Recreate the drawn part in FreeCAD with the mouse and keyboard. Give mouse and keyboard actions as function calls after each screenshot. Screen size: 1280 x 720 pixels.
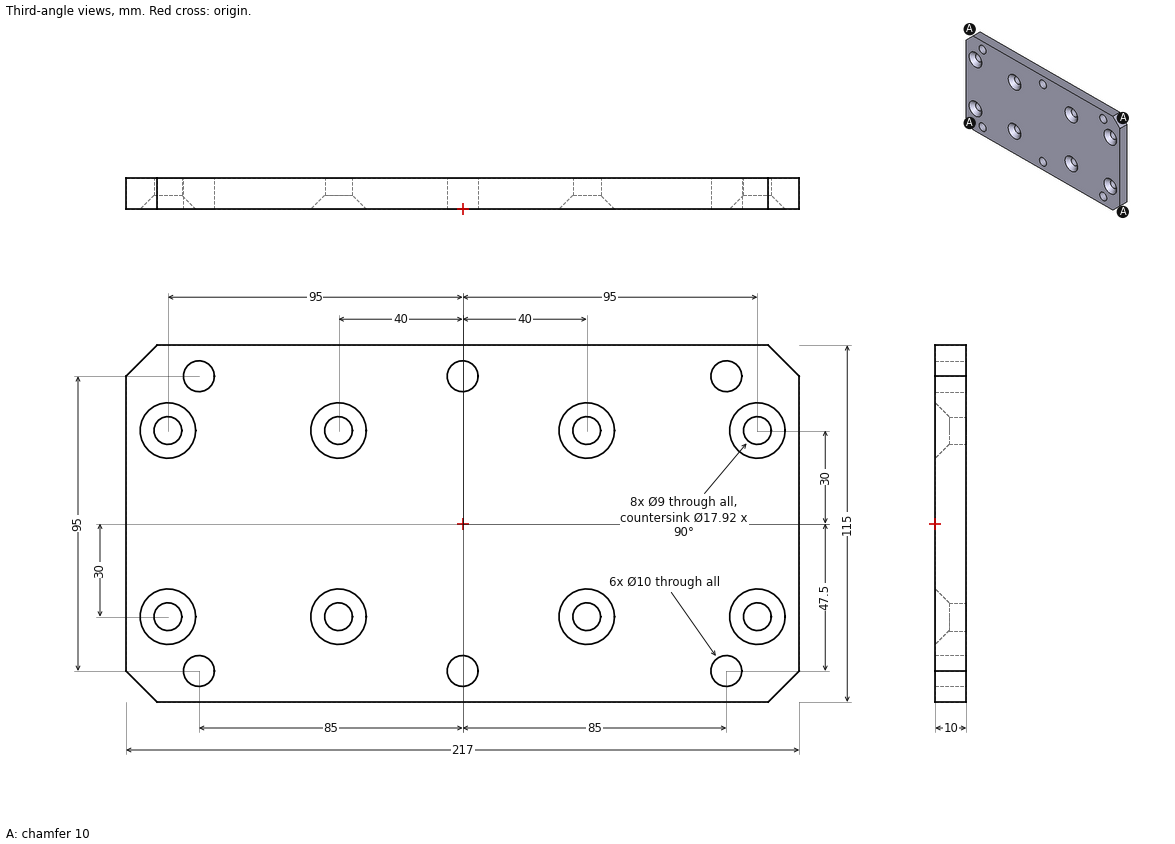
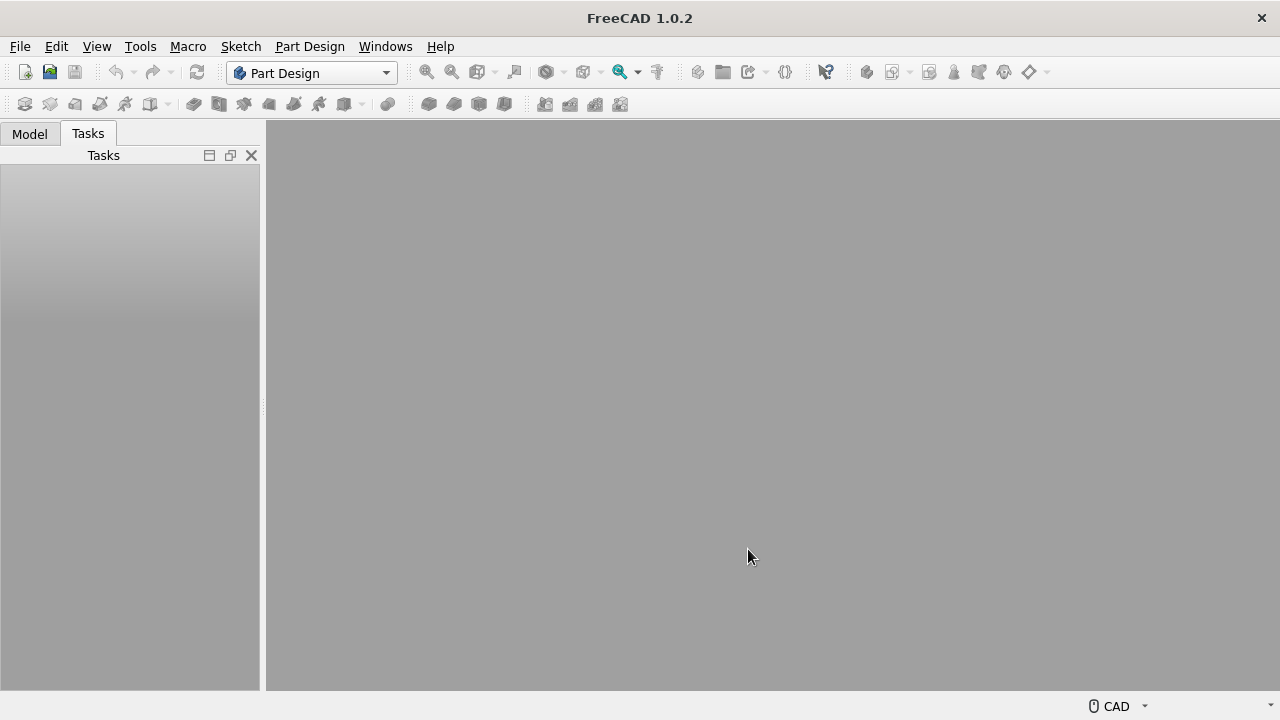
click(25, 72)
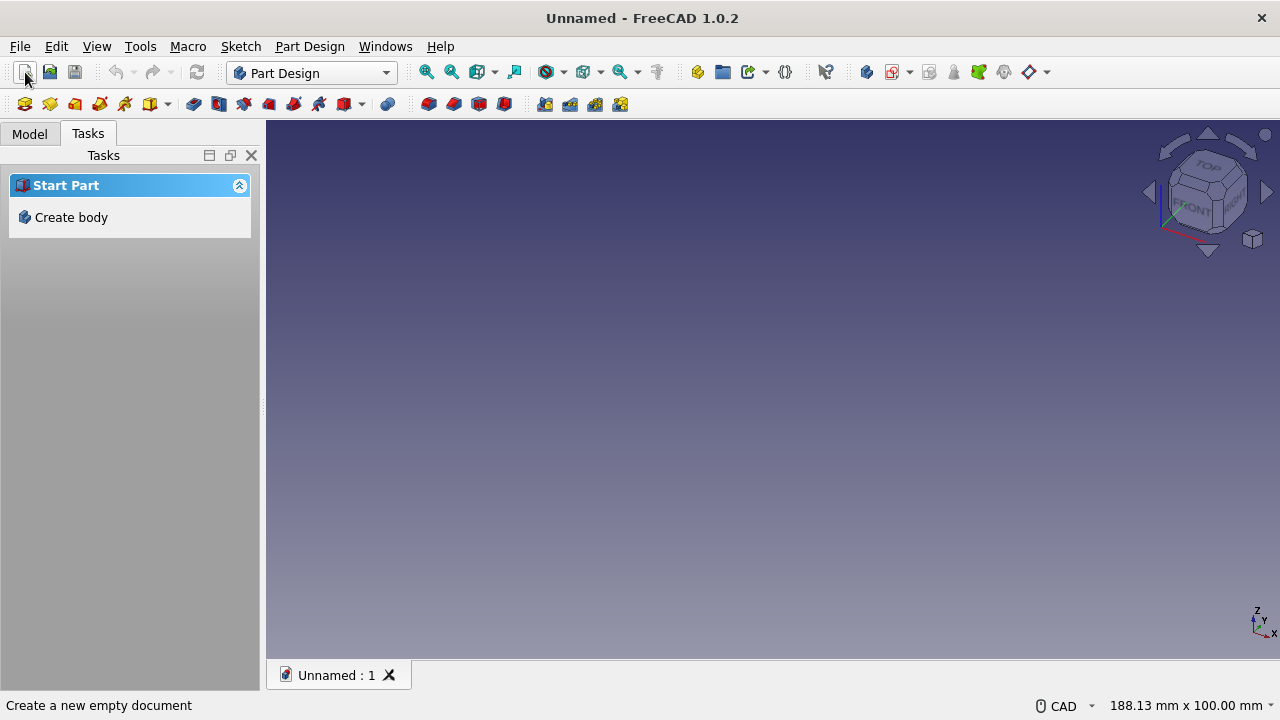
click(892, 72)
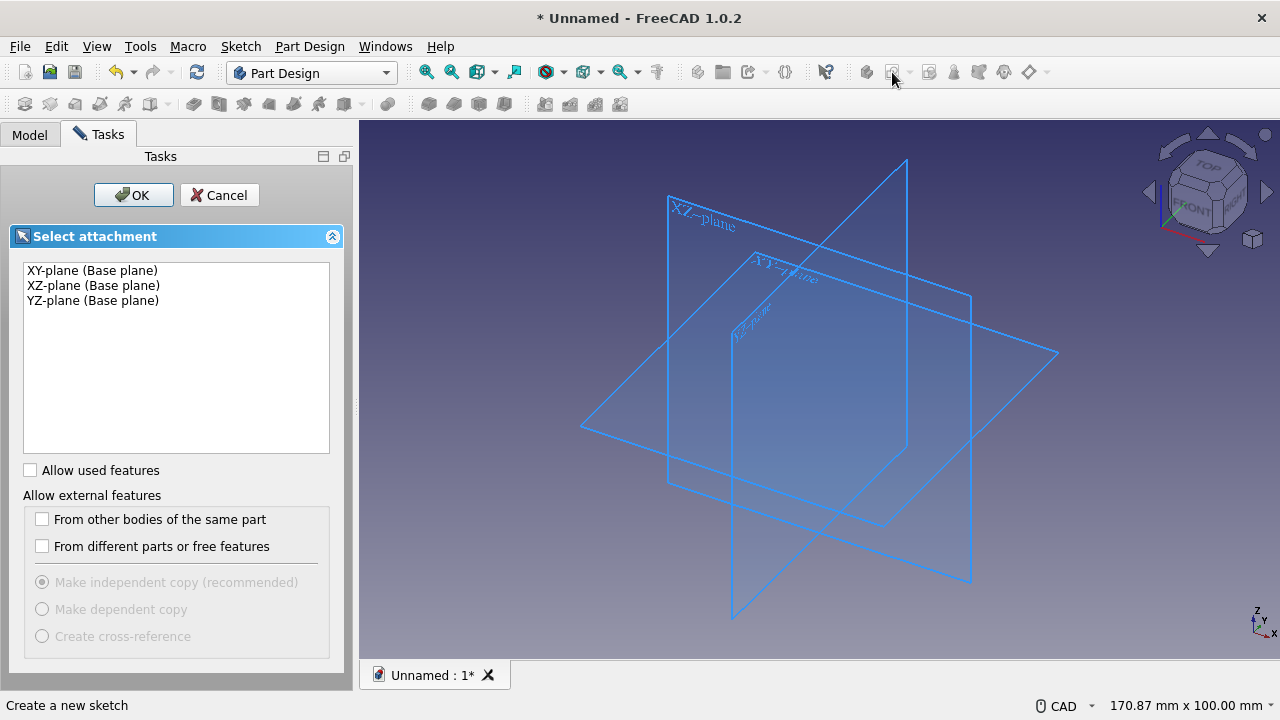
click(84, 286)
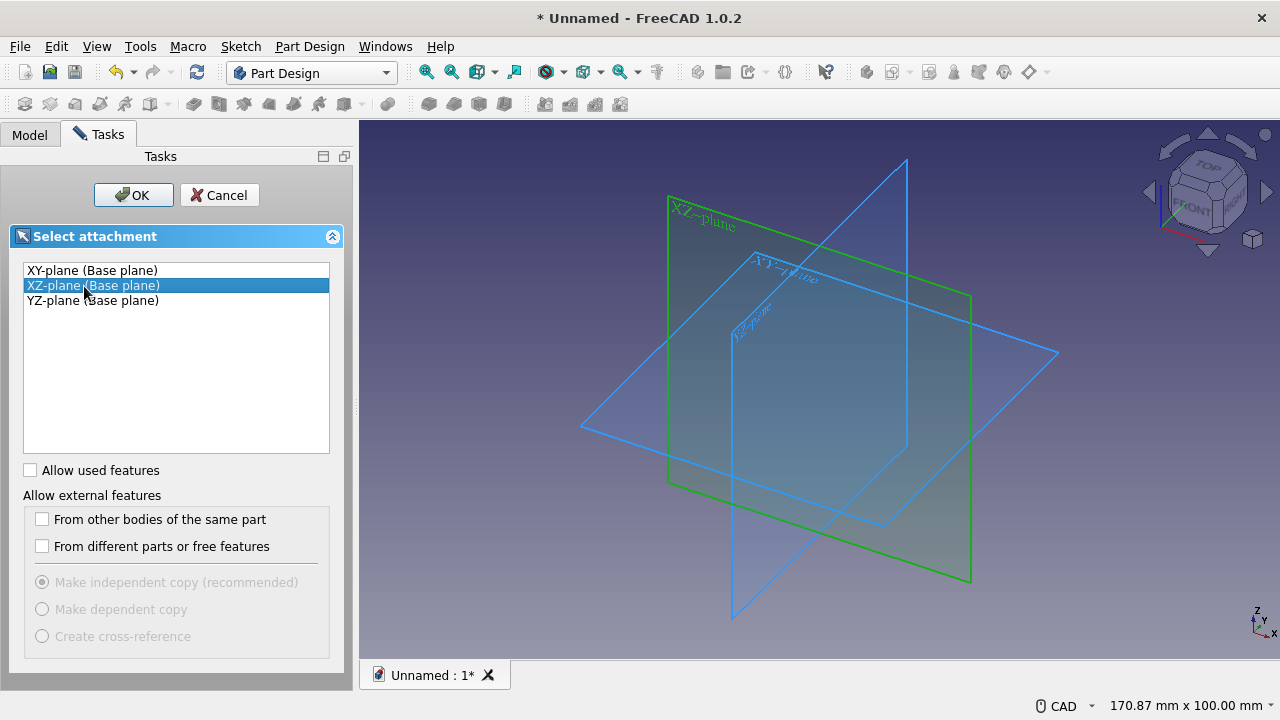
click(134, 195)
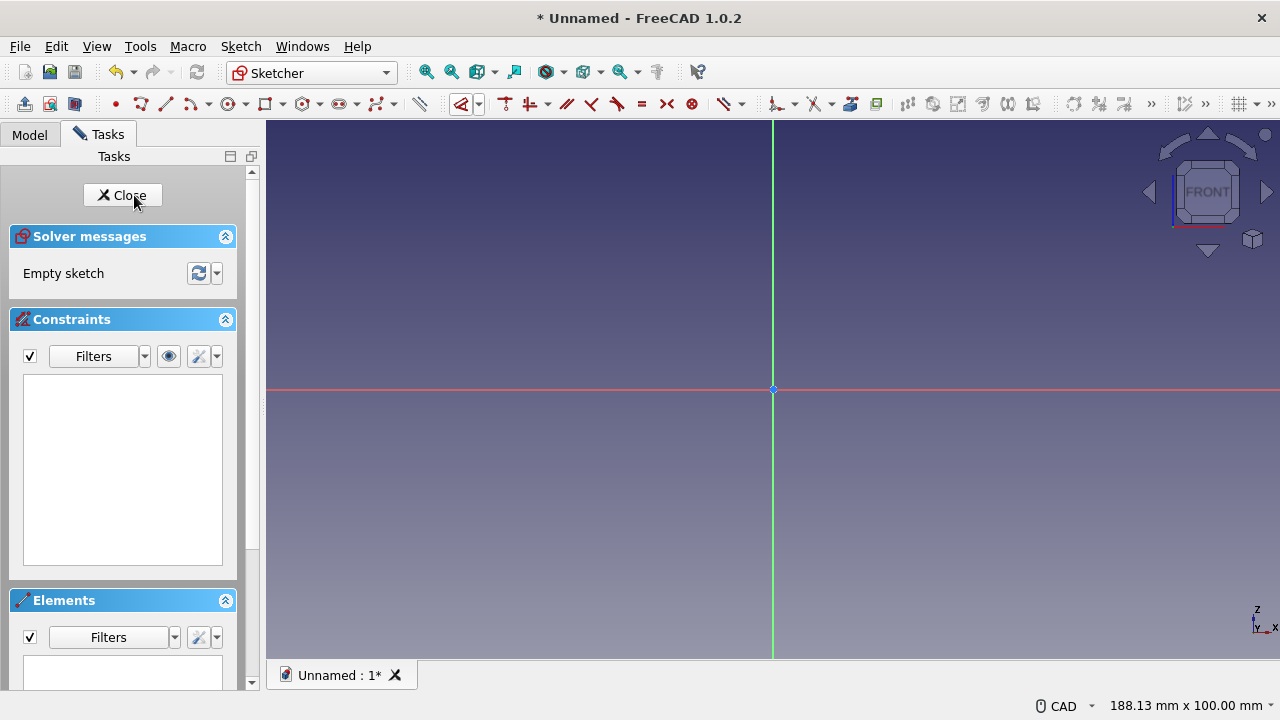
scroll(649, 390, down, 4)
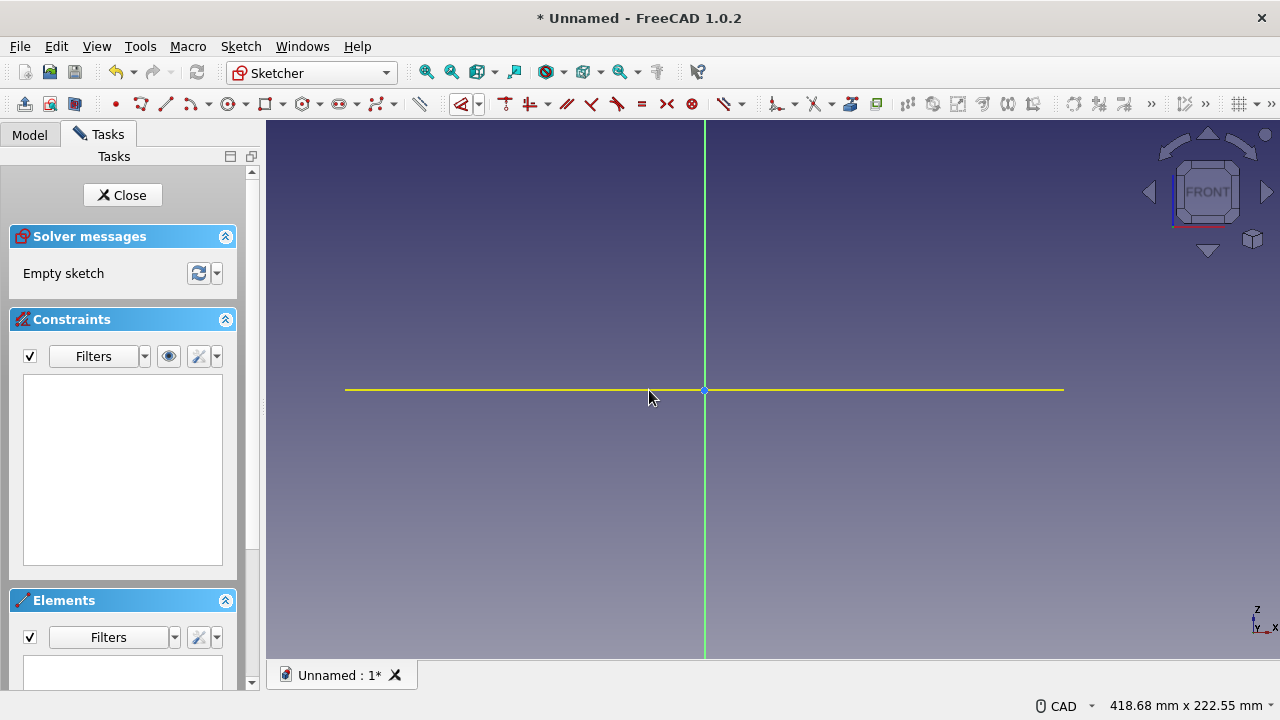
click(282, 104)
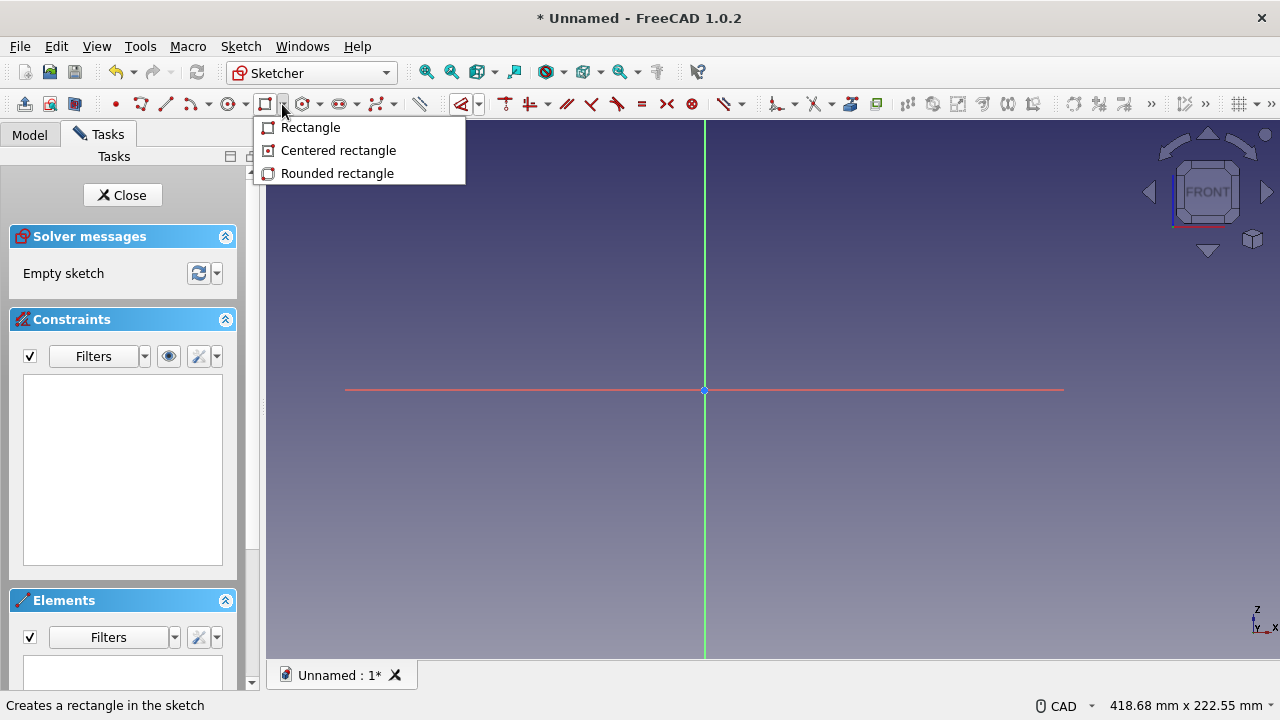
click(360, 150)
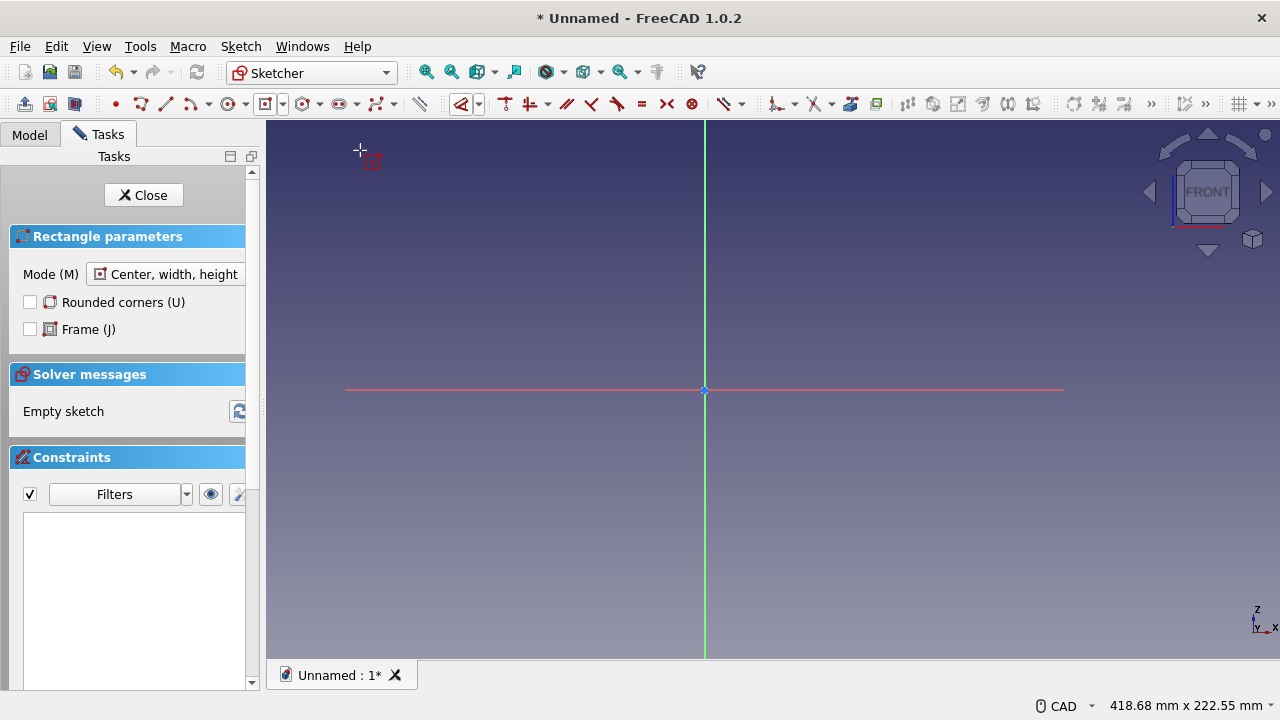
click(705, 390)
click(968, 251)
key(Escape)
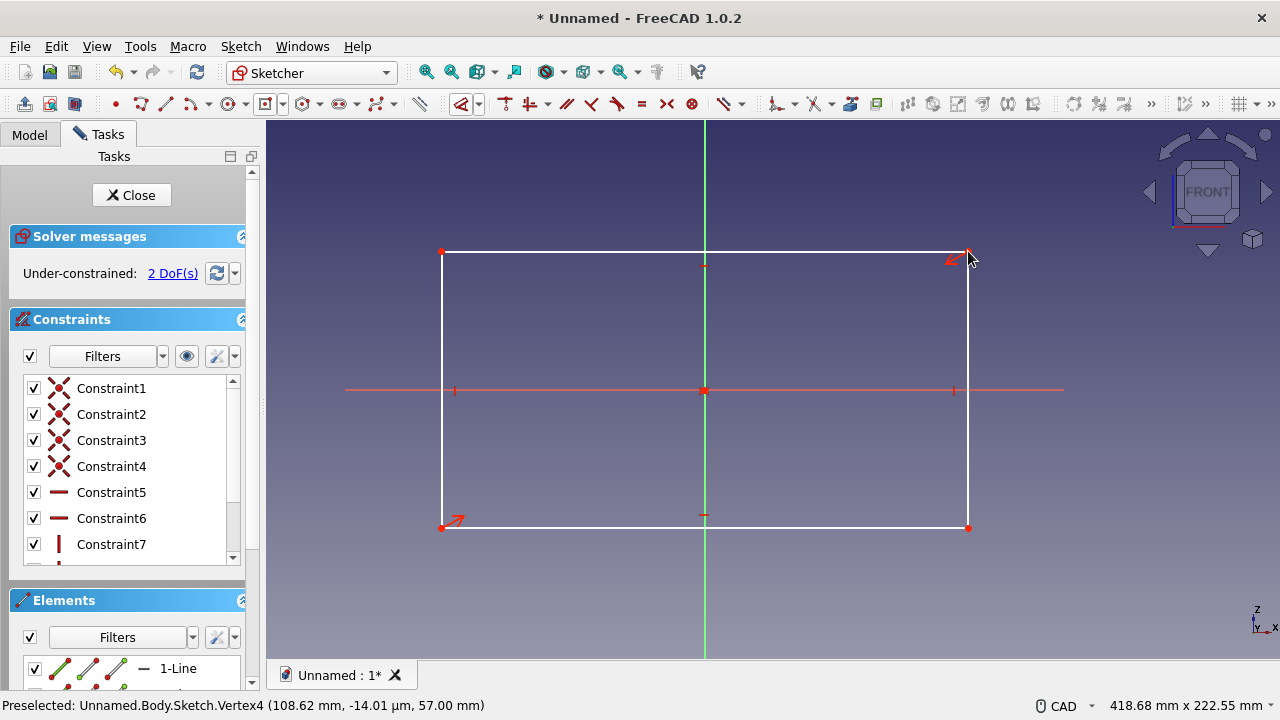
click(460, 104)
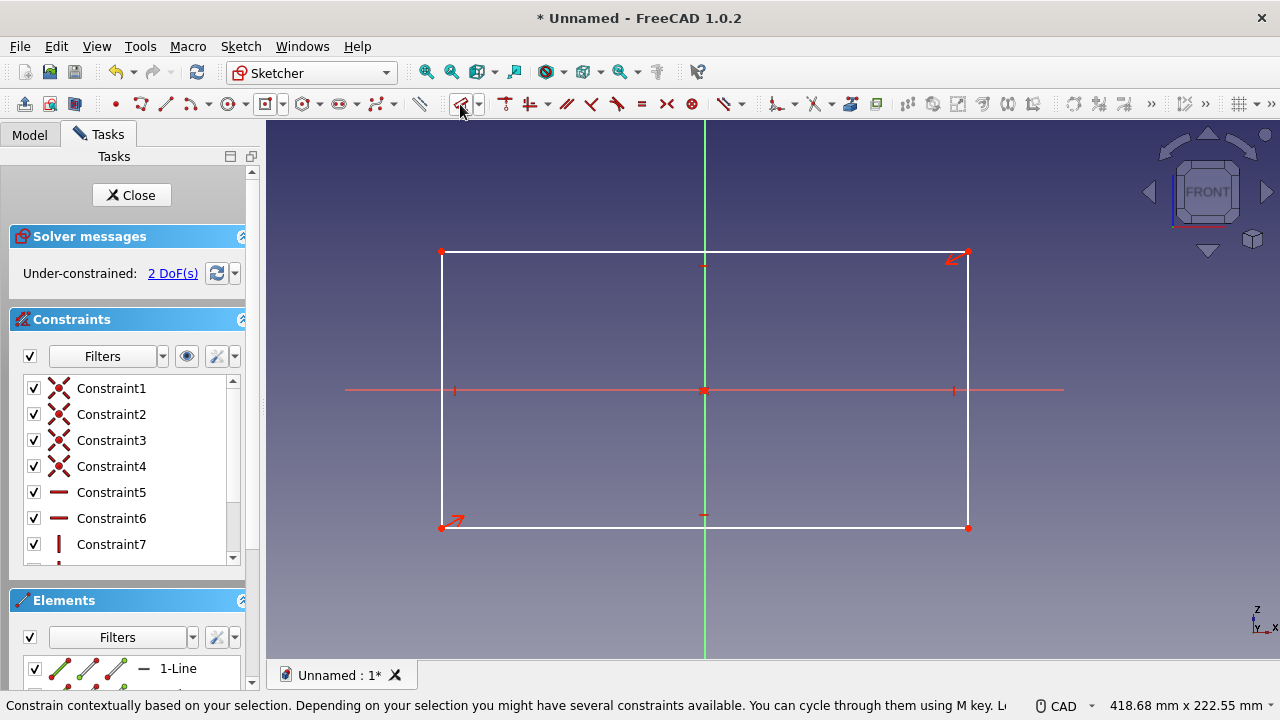
click(600, 528)
click(584, 562)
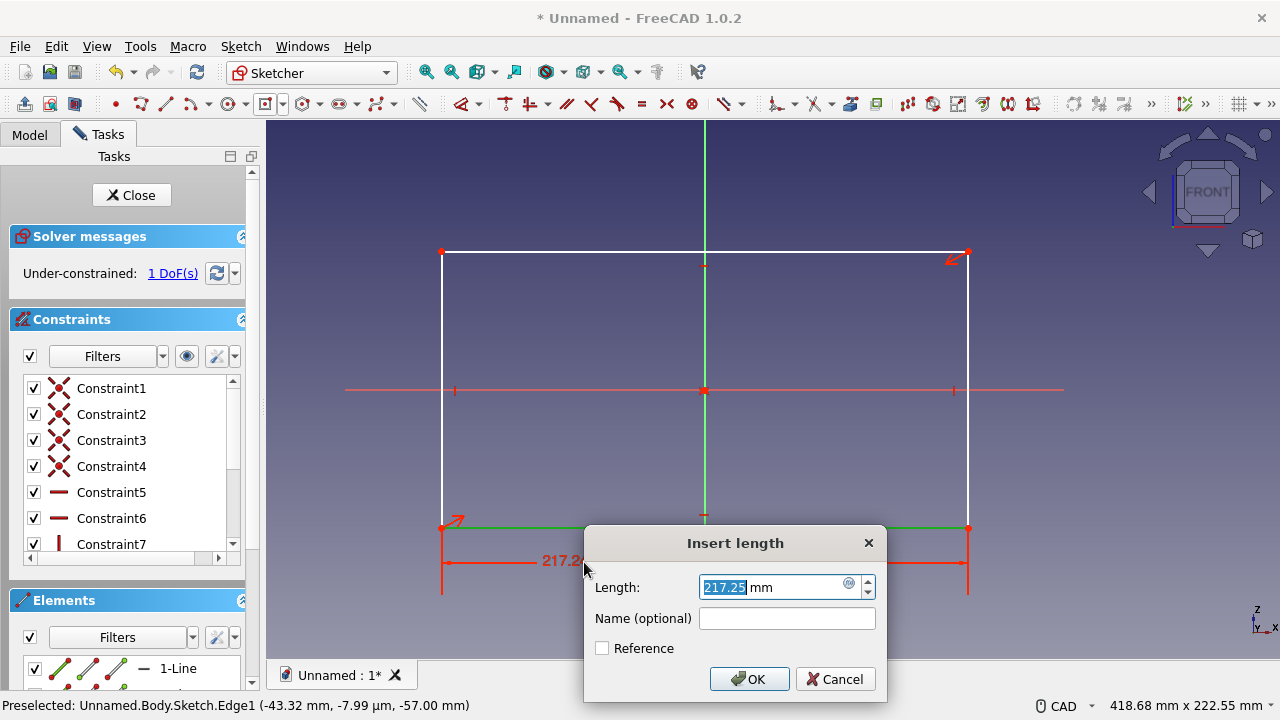
text(217)
key(Return)